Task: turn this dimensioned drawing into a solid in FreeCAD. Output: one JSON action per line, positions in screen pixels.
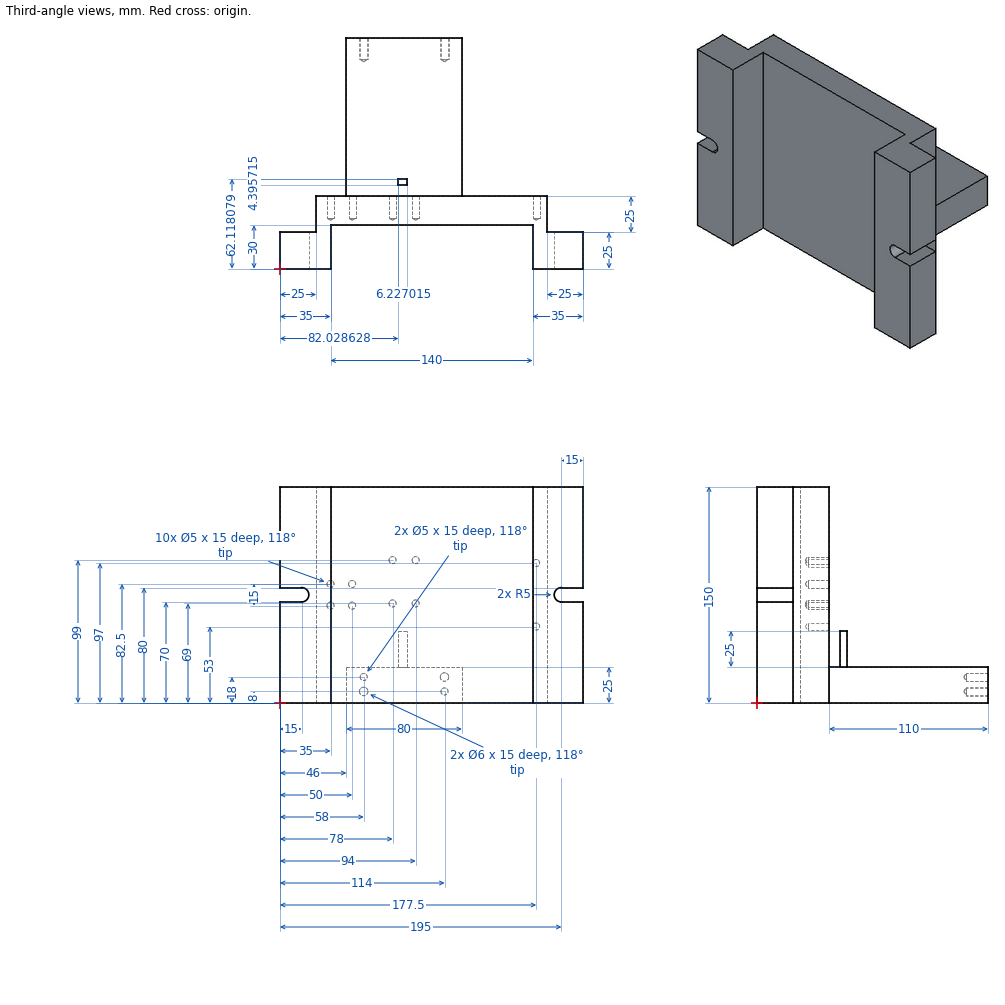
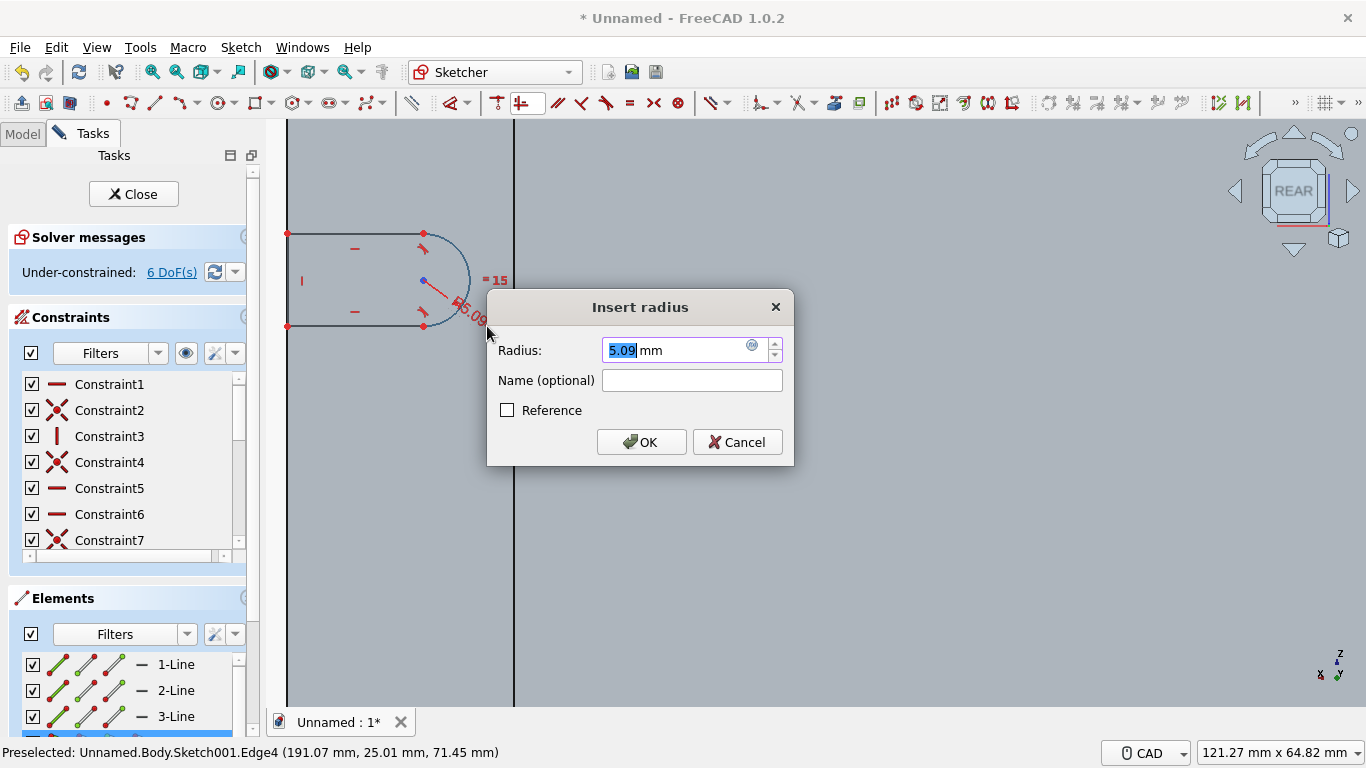
{"action": "type", "text": "5"}
{"action": "key", "text": "Return"}
{"action": "key", "text": "Escape"}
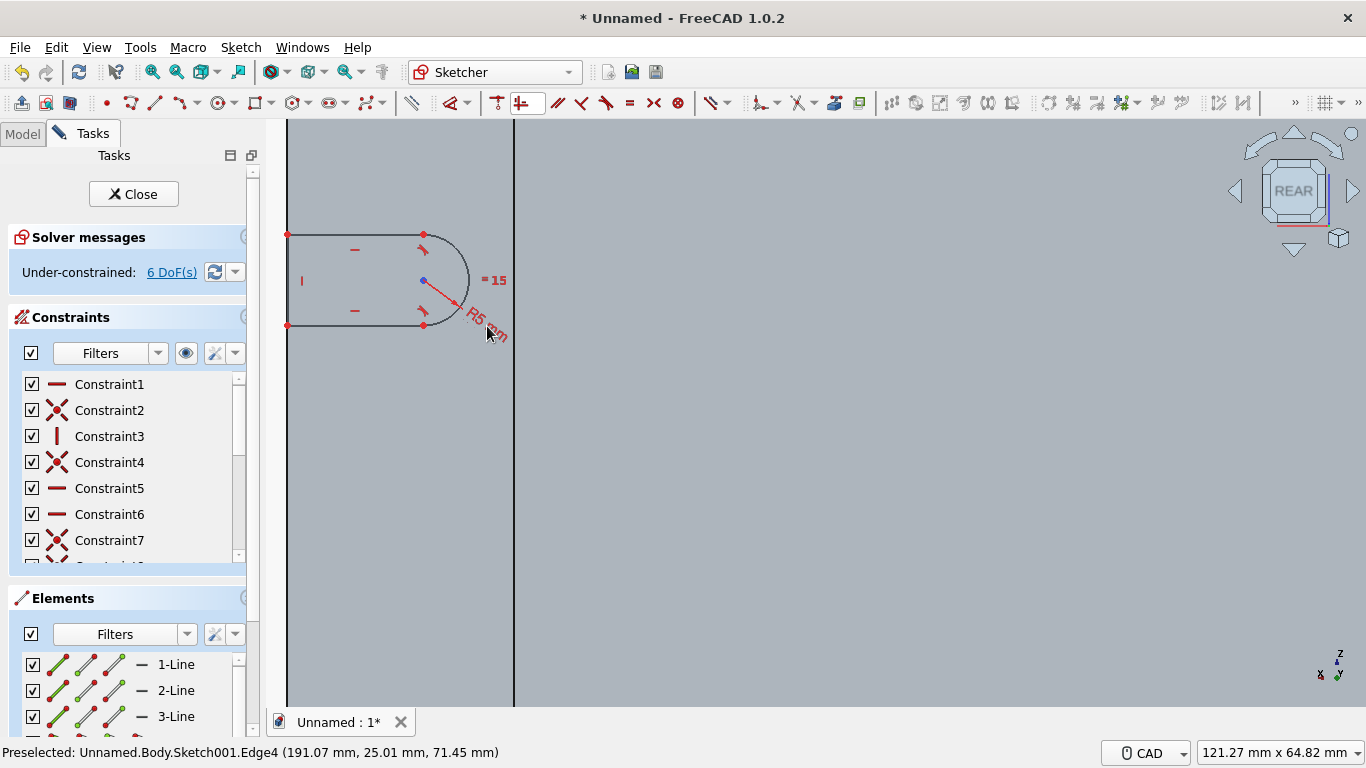
{"action": "scroll", "coordinate": [461, 307], "scroll_direction": "down", "scroll_amount": 5}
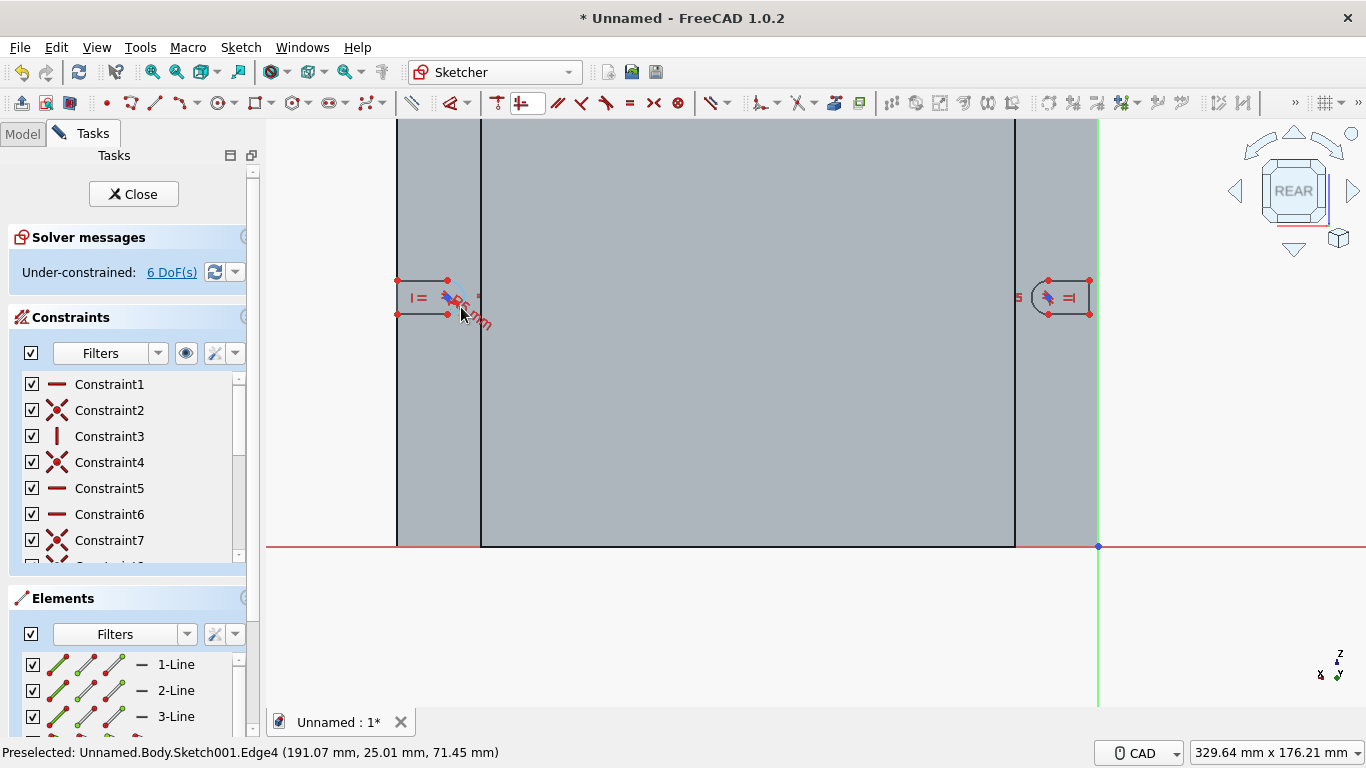
{"action": "left_click", "coordinate": [1089, 314]}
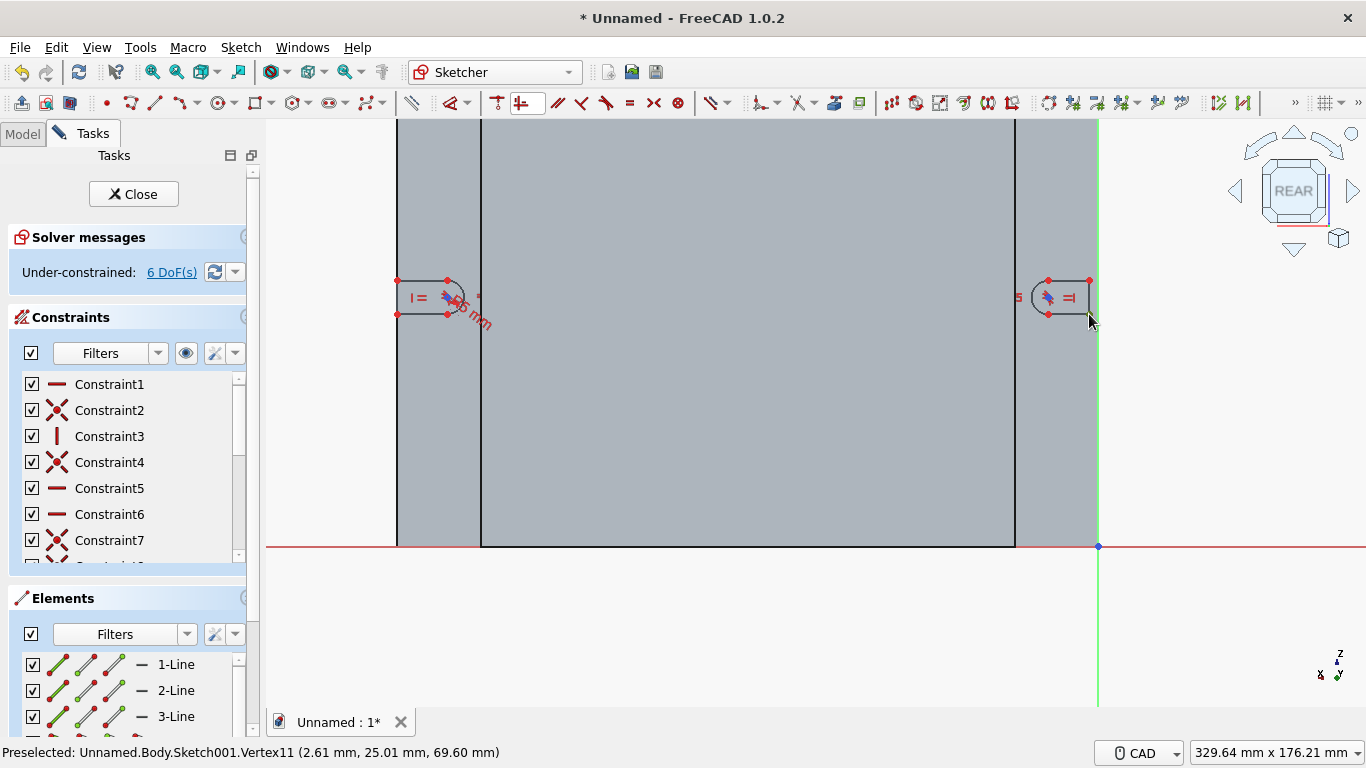
{"action": "left_click", "coordinate": [1098, 641]}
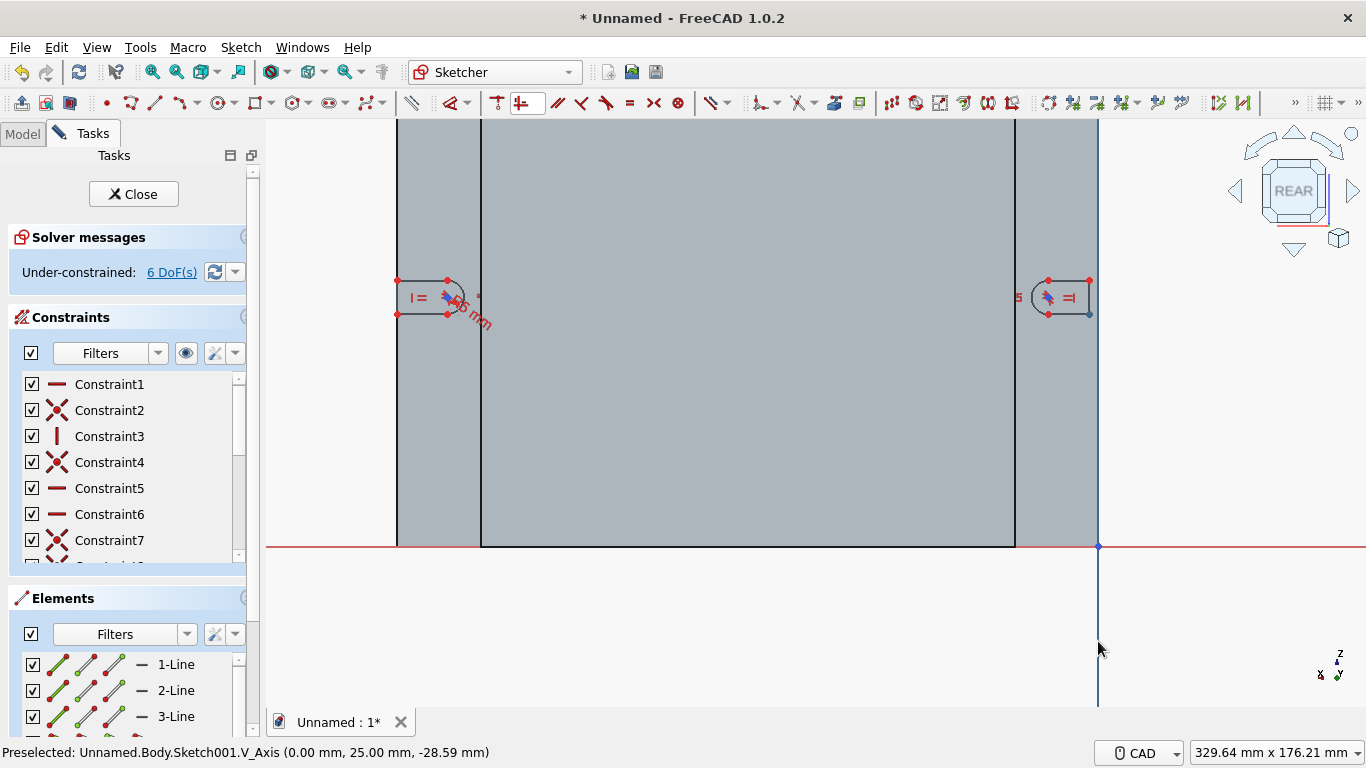
{"action": "left_click", "coordinate": [498, 104]}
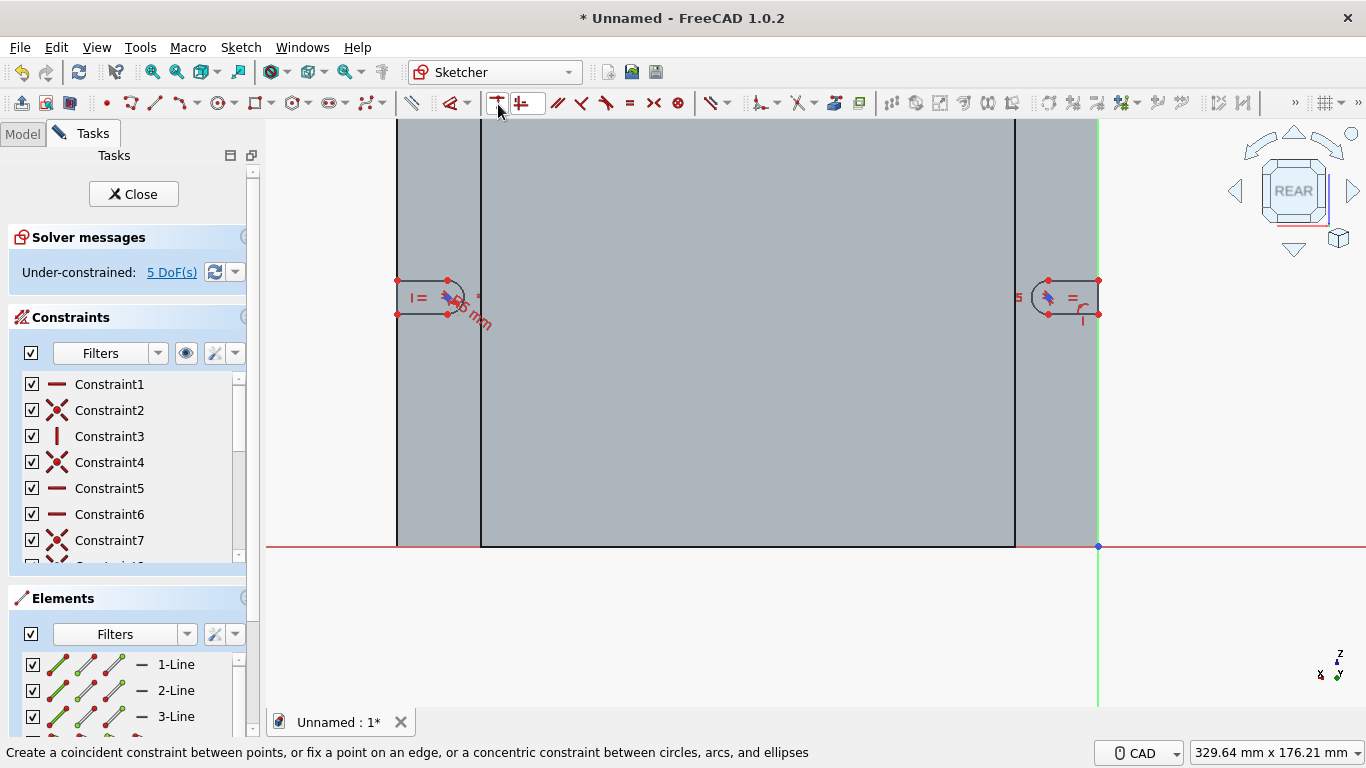
{"action": "key", "text": "d"}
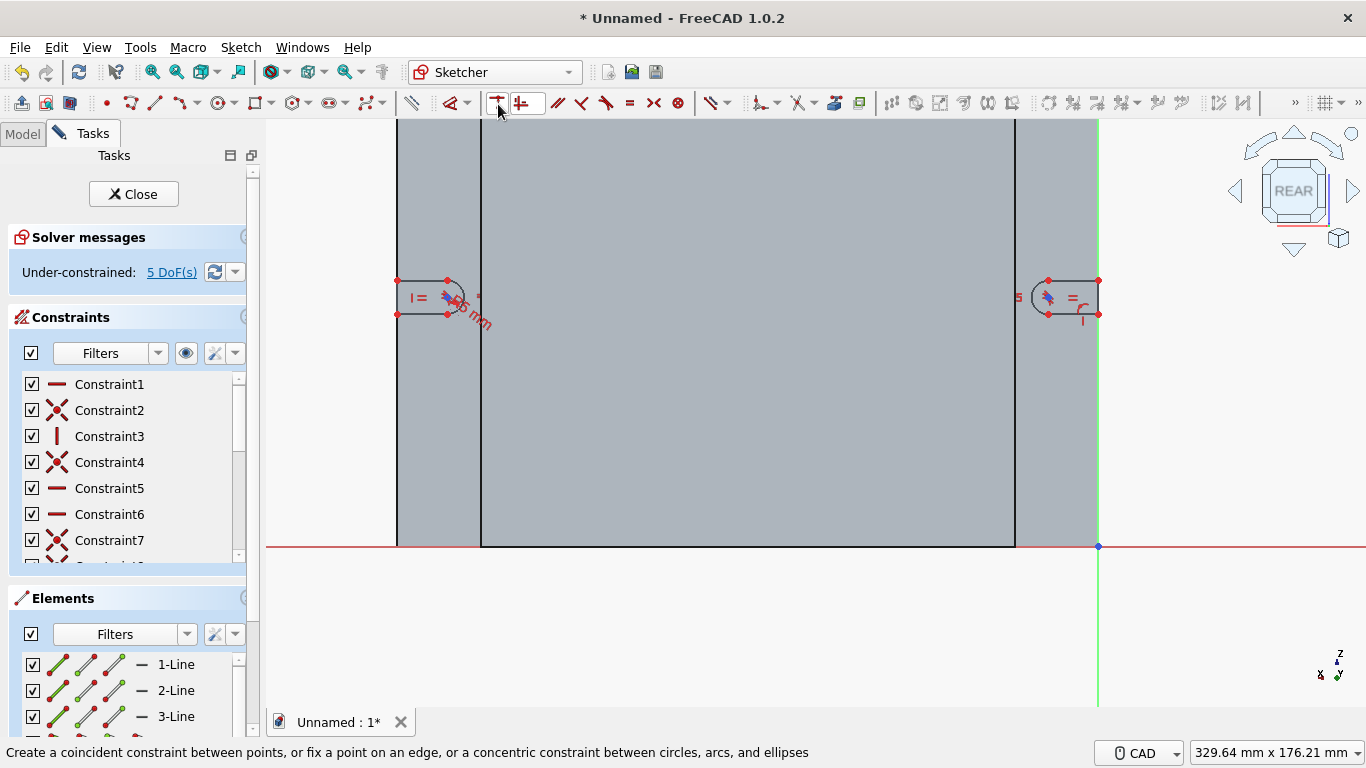
{"action": "left_click", "coordinate": [432, 281]}
{"action": "left_click", "coordinate": [422, 247]}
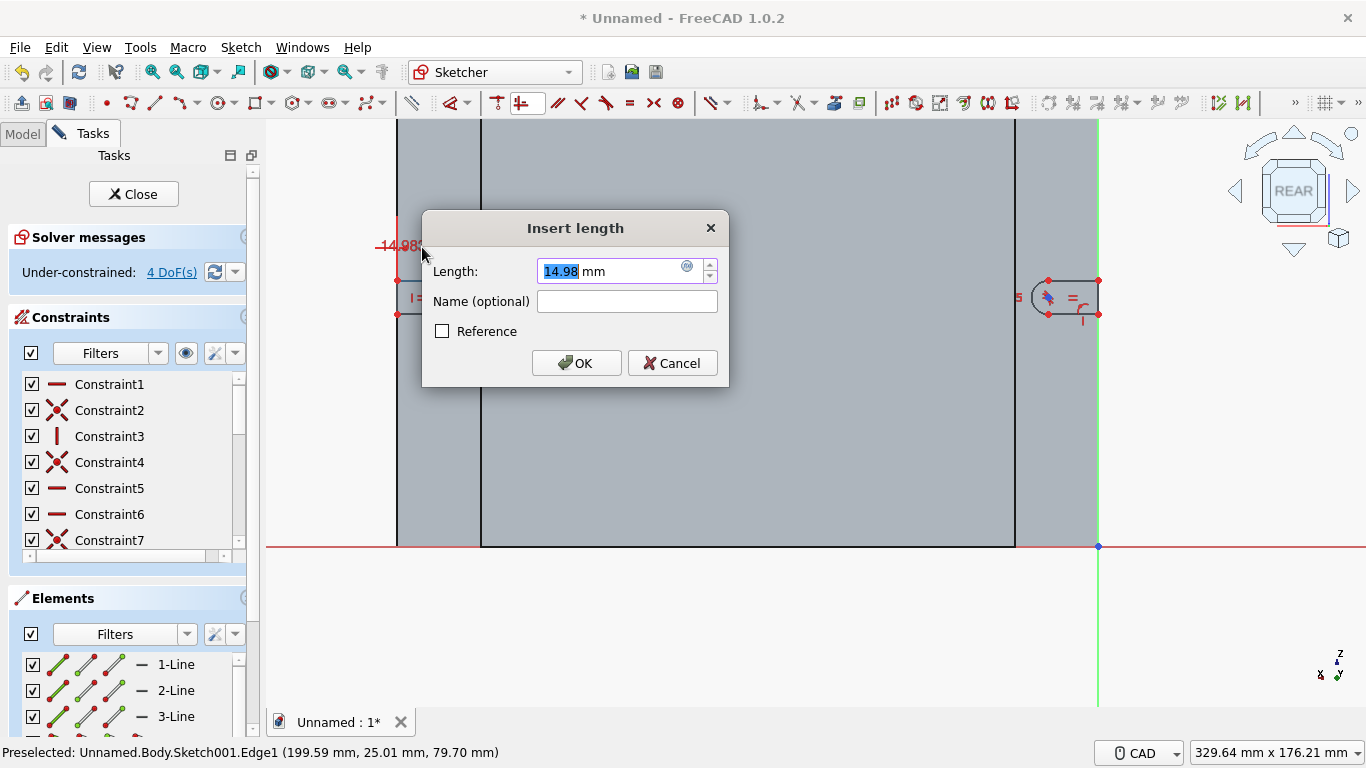
{"action": "type", "text": "15"}
{"action": "key", "text": "Return"}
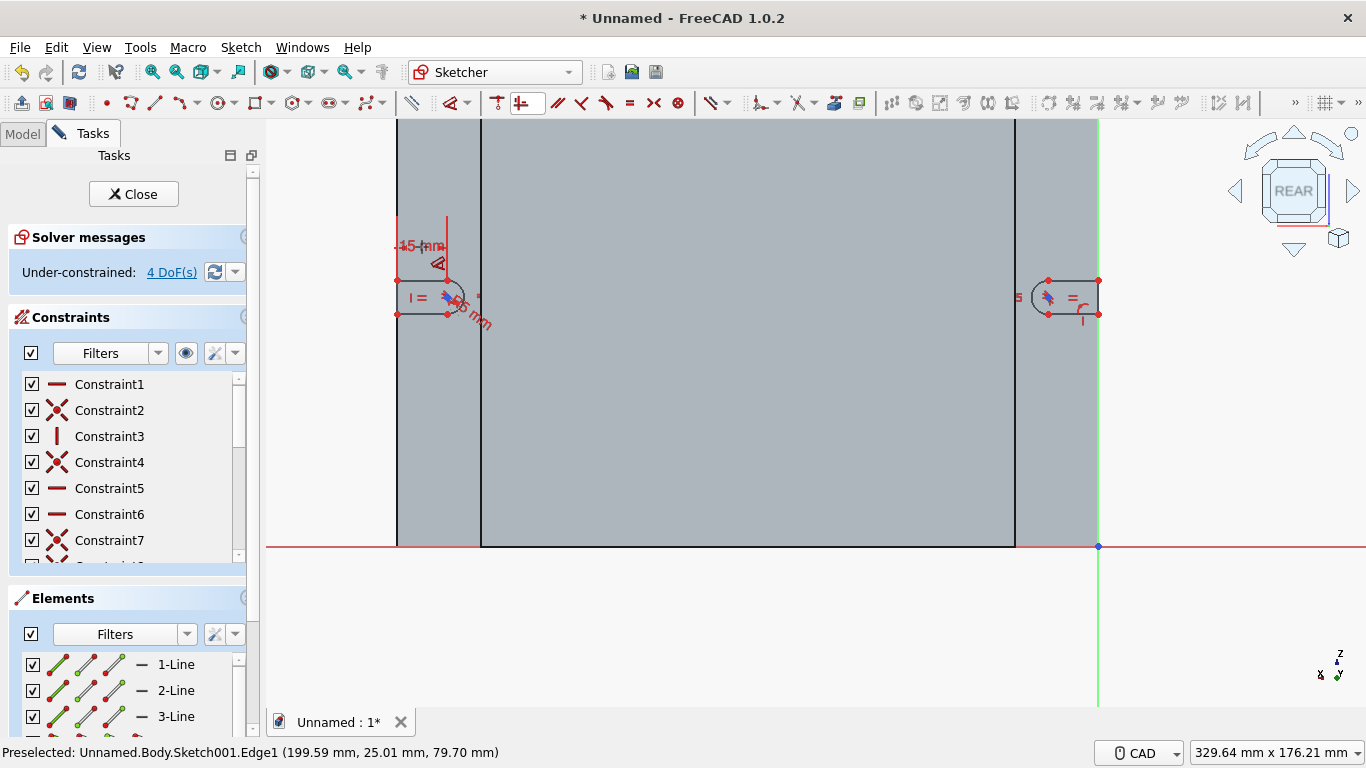
{"action": "left_click", "coordinate": [1063, 314]}
{"action": "left_click", "coordinate": [1073, 348]}